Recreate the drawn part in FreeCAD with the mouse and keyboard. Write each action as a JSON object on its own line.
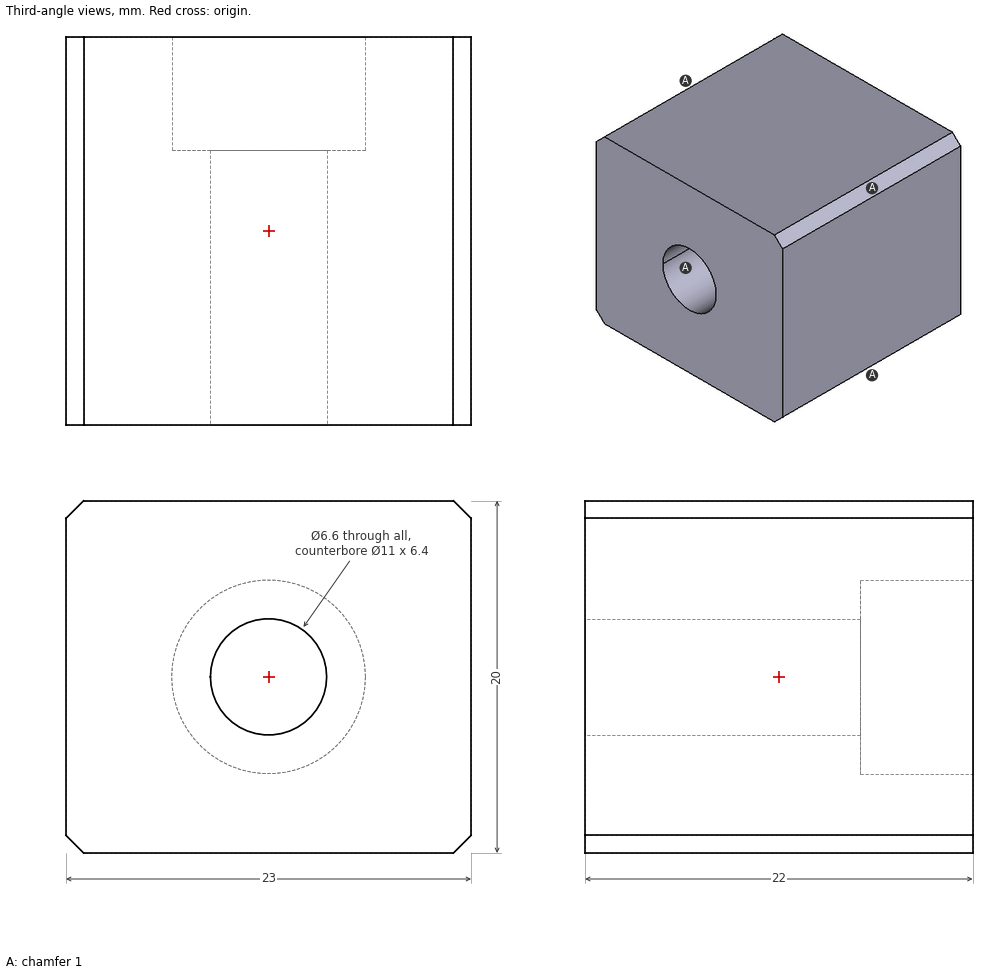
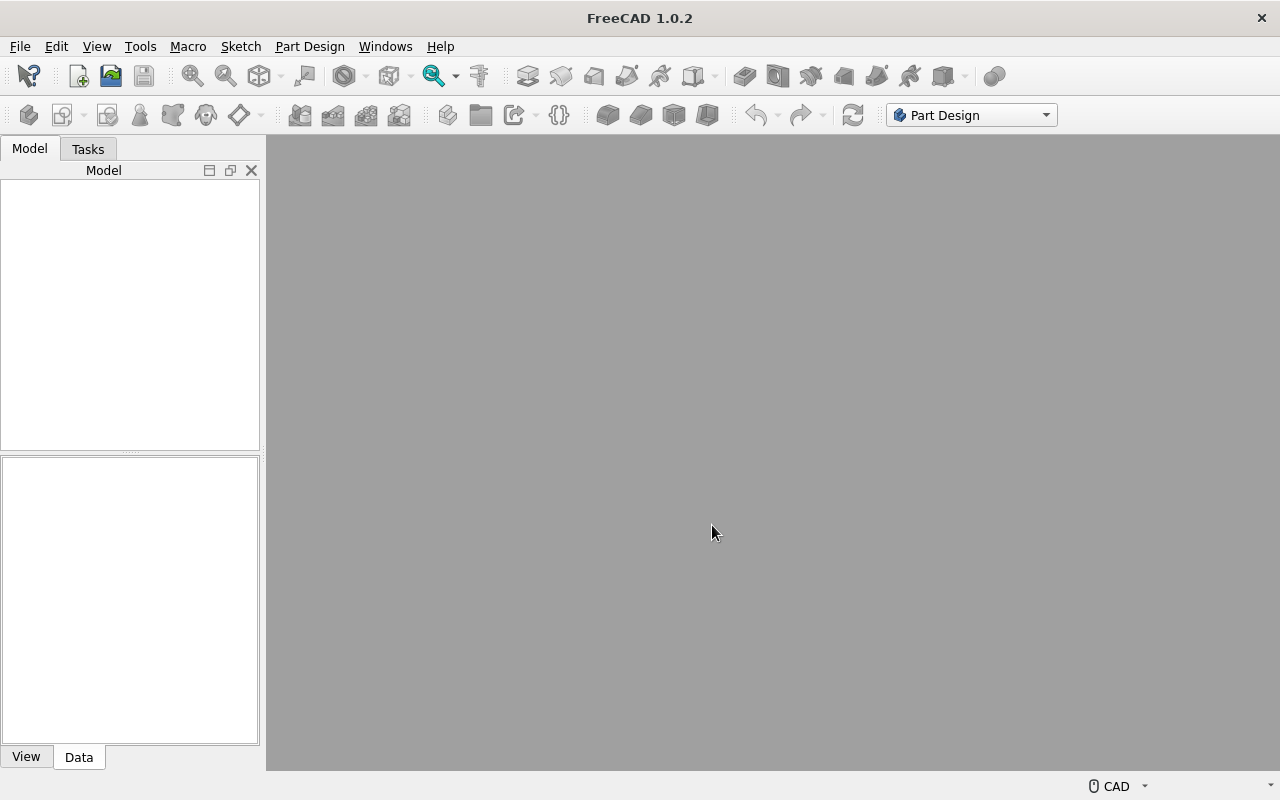
{"action": "left_click", "coordinate": [78, 76]}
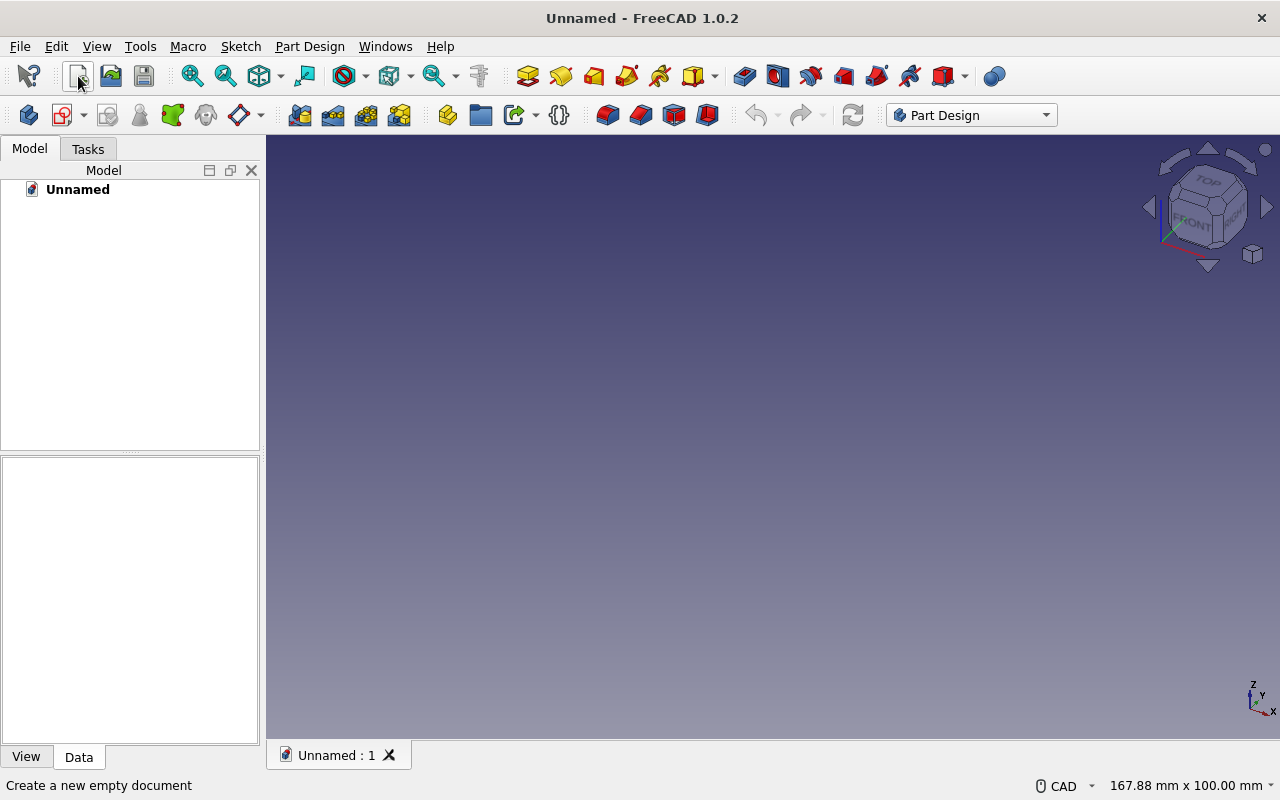
{"action": "left_click", "coordinate": [62, 116]}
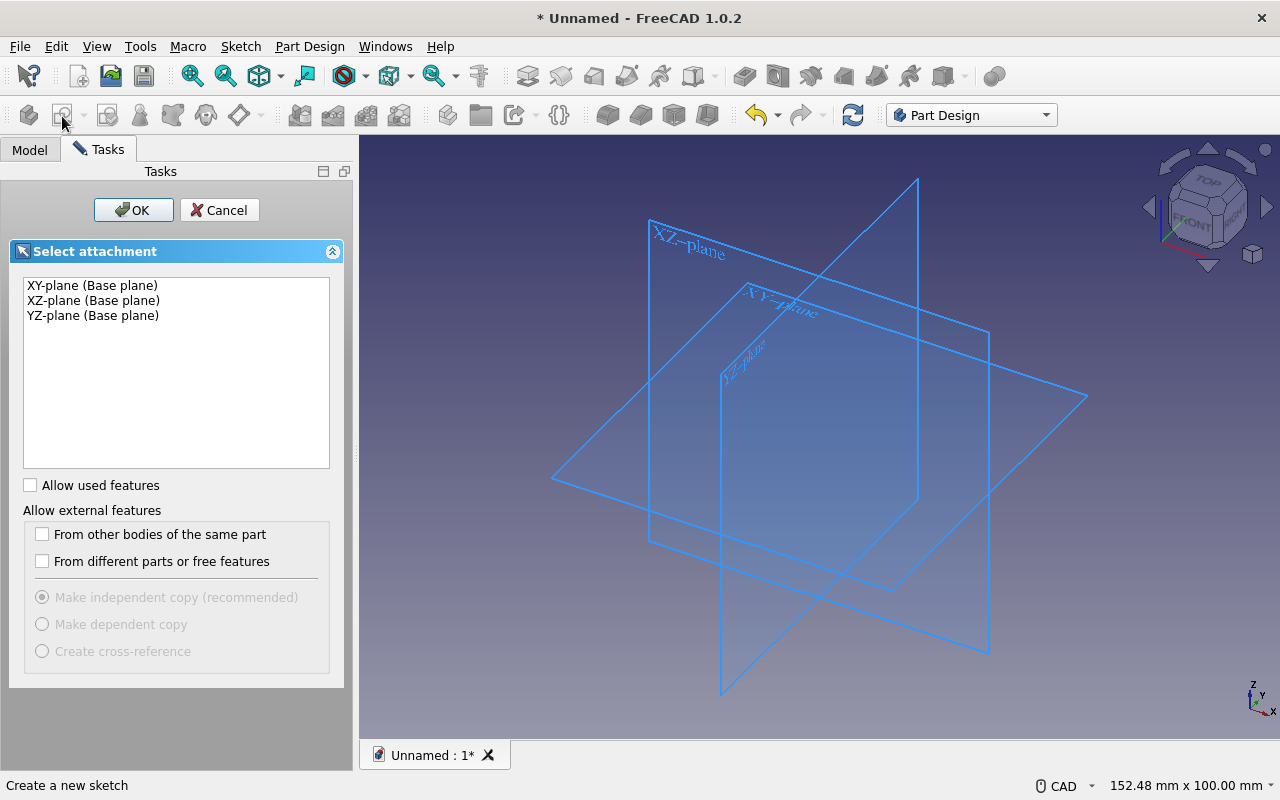
{"action": "left_click", "coordinate": [84, 300]}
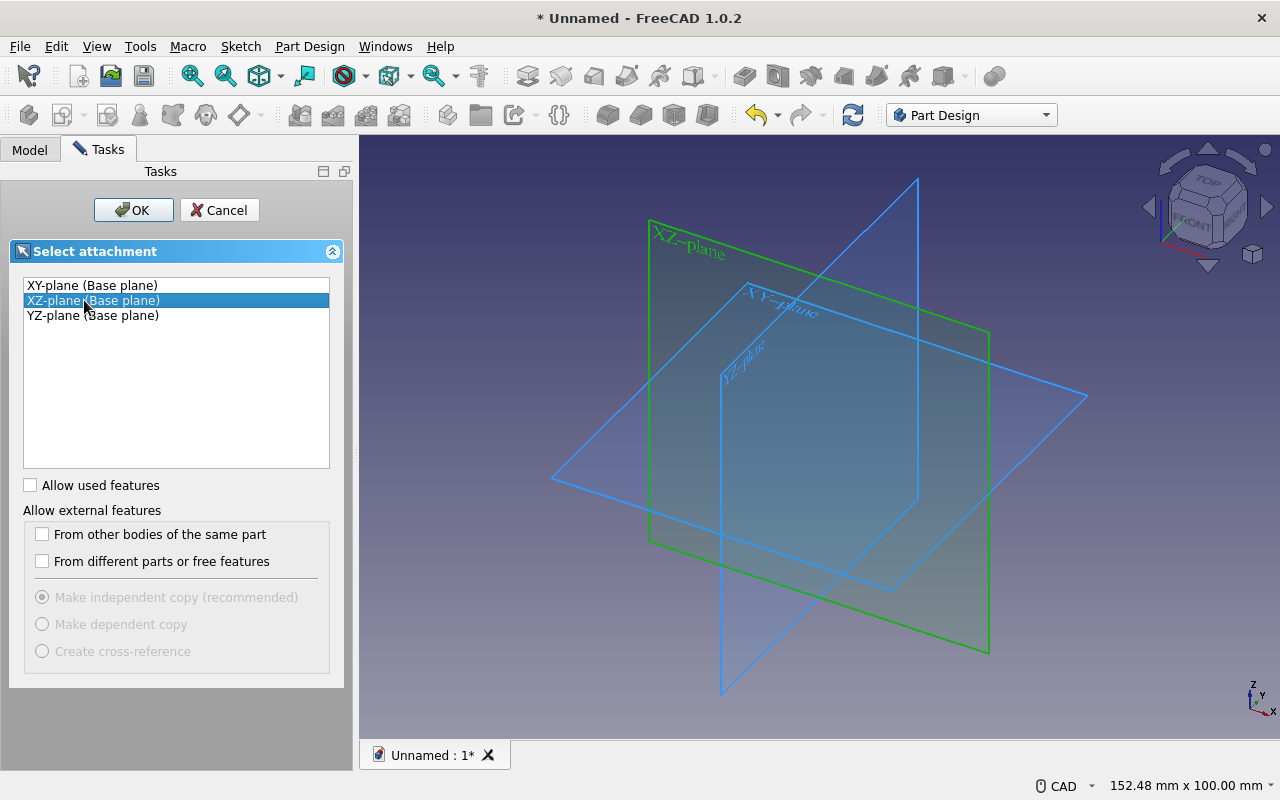
{"action": "left_click", "coordinate": [134, 210]}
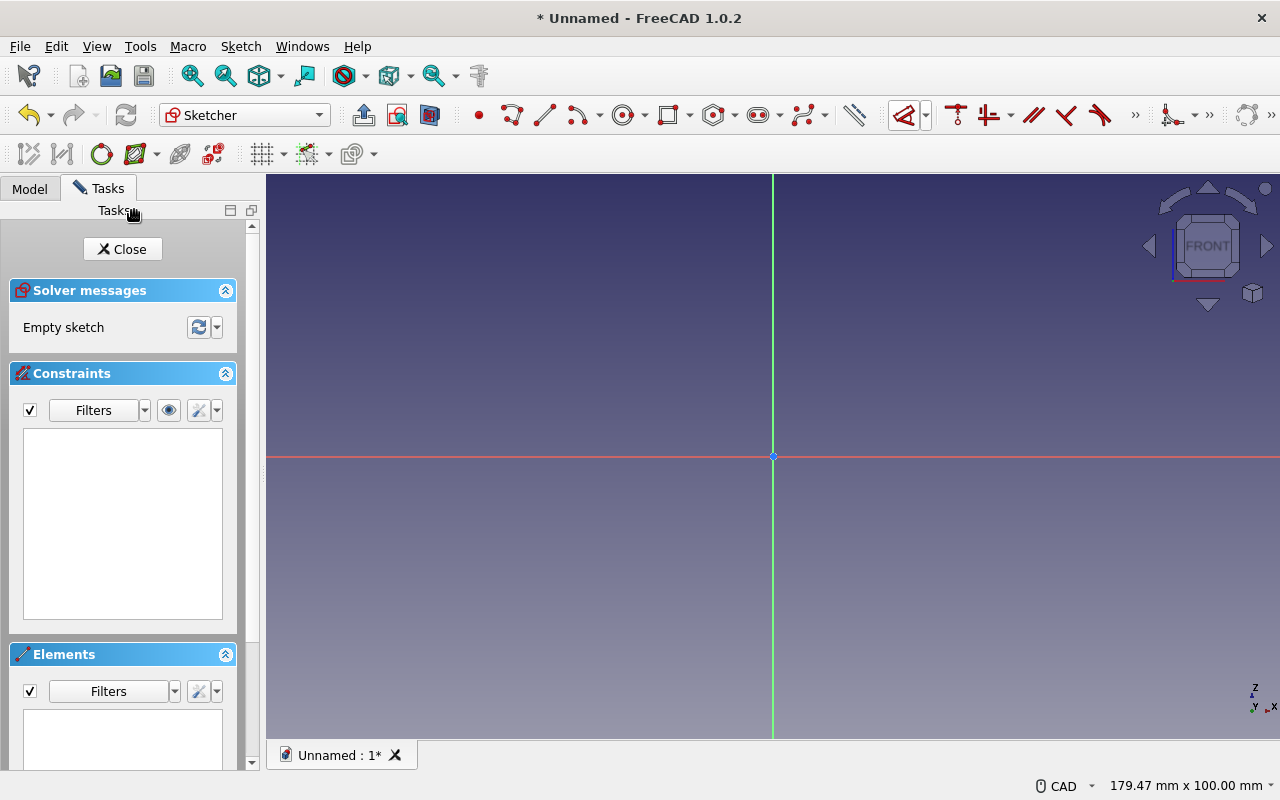
{"action": "scroll", "coordinate": [803, 456], "scroll_direction": "up", "scroll_amount": 6}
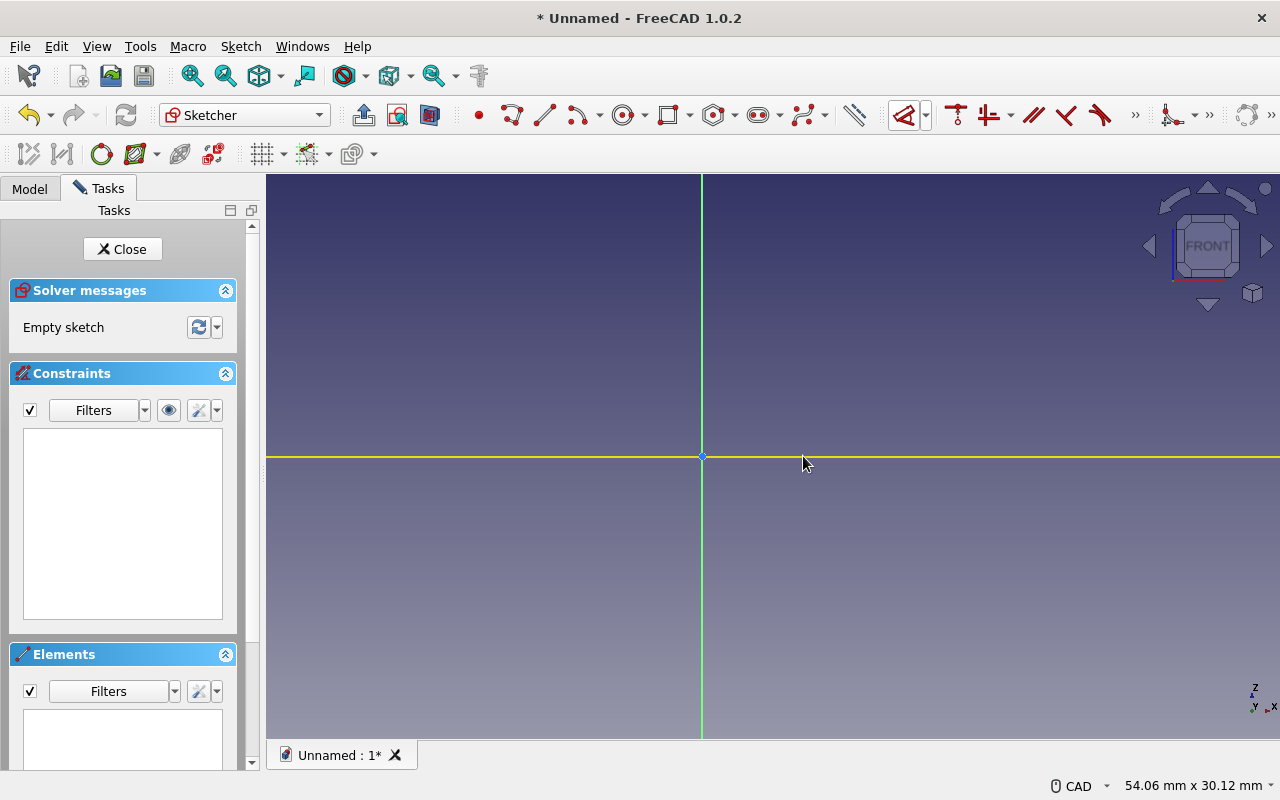
{"action": "key", "text": "g v"}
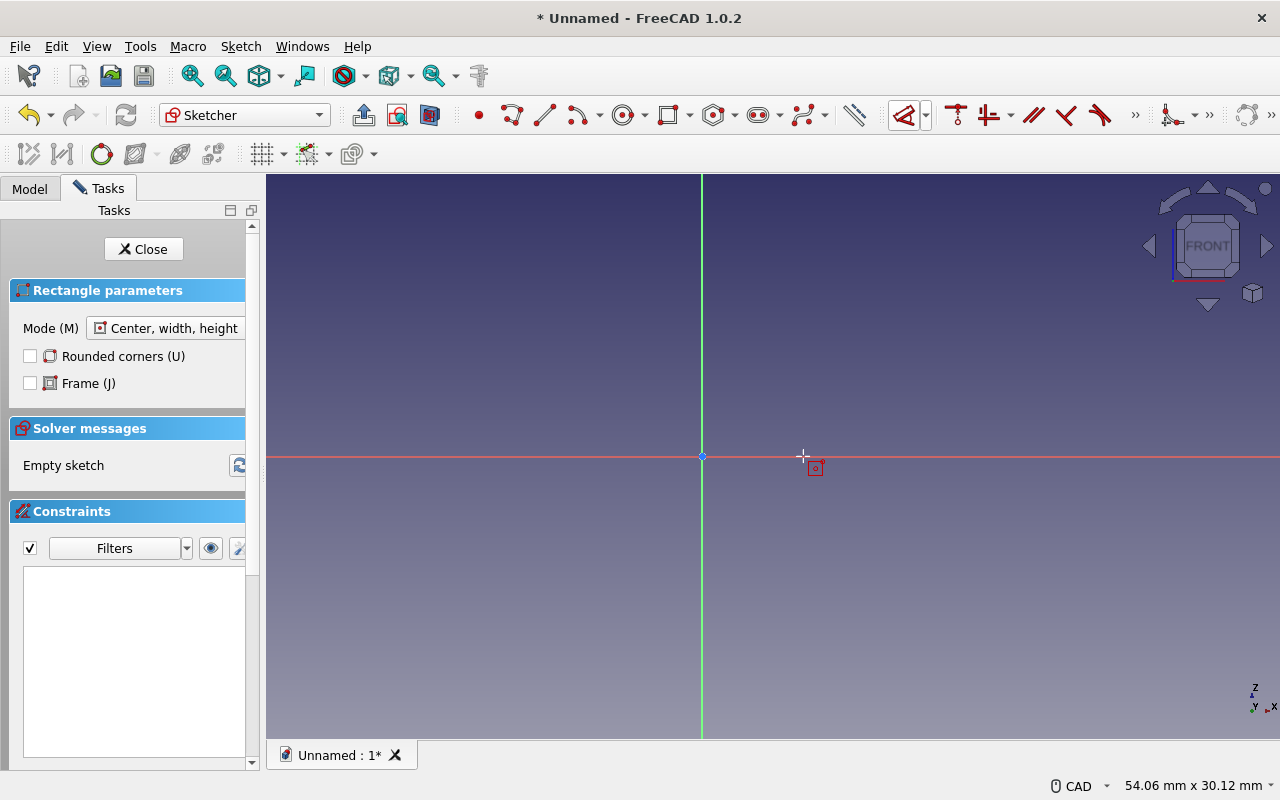
{"action": "left_click", "coordinate": [702, 456]}
{"action": "left_click", "coordinate": [918, 269]}
{"action": "key", "text": "Escape"}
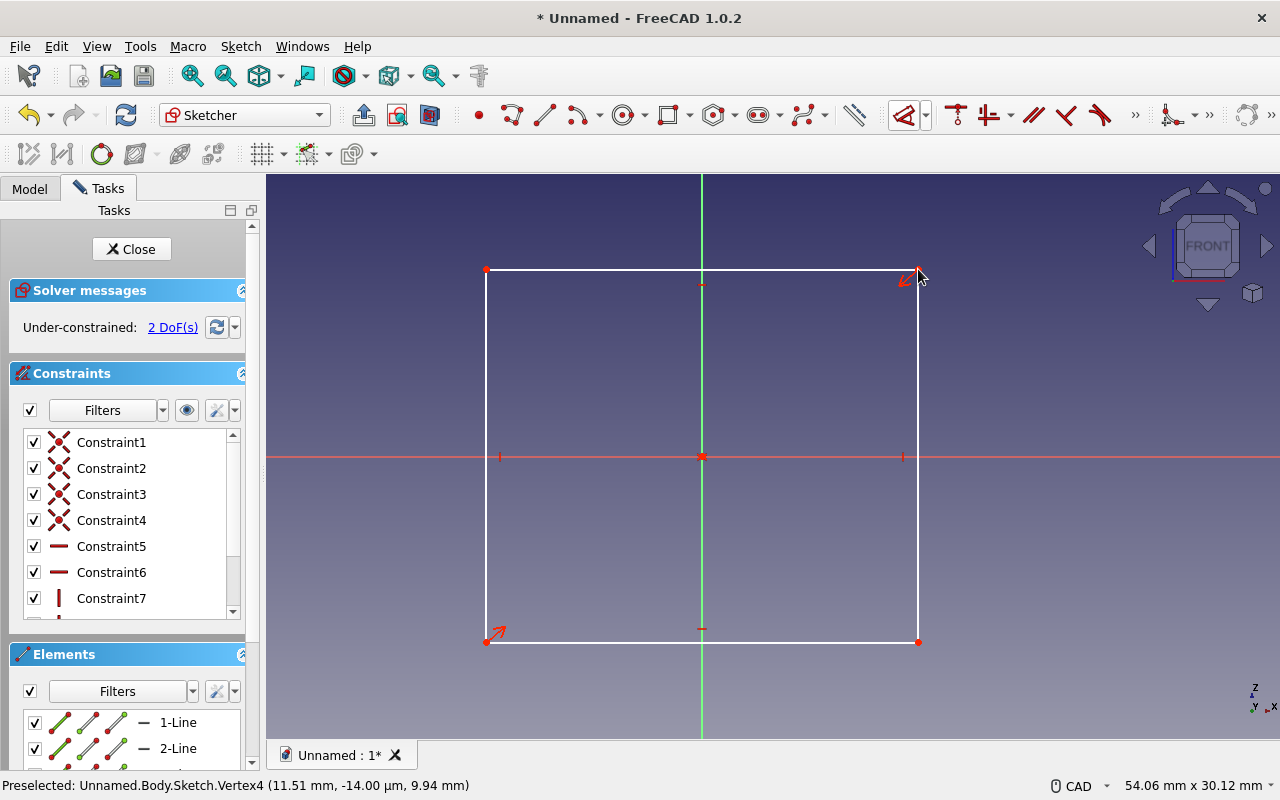
{"action": "key", "text": "d"}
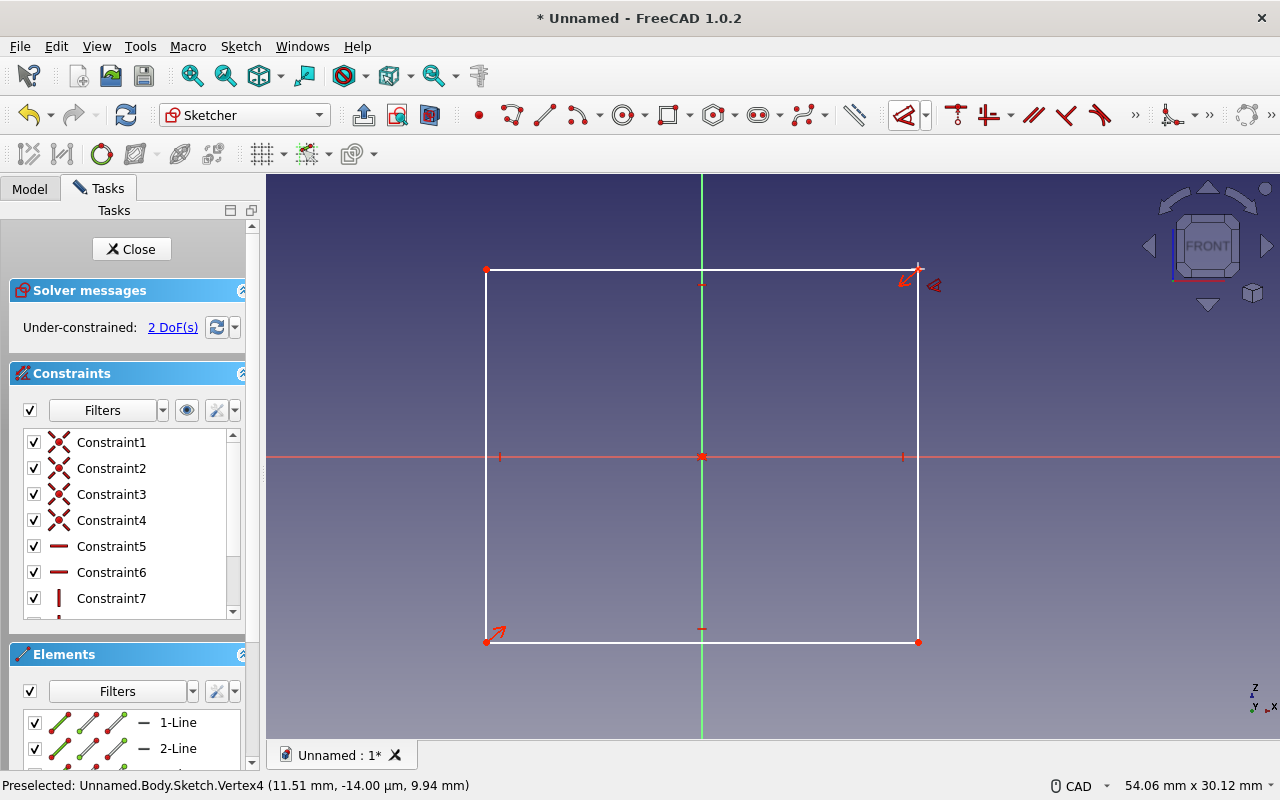
{"action": "left_click", "coordinate": [616, 643]}
{"action": "left_click", "coordinate": [603, 677]}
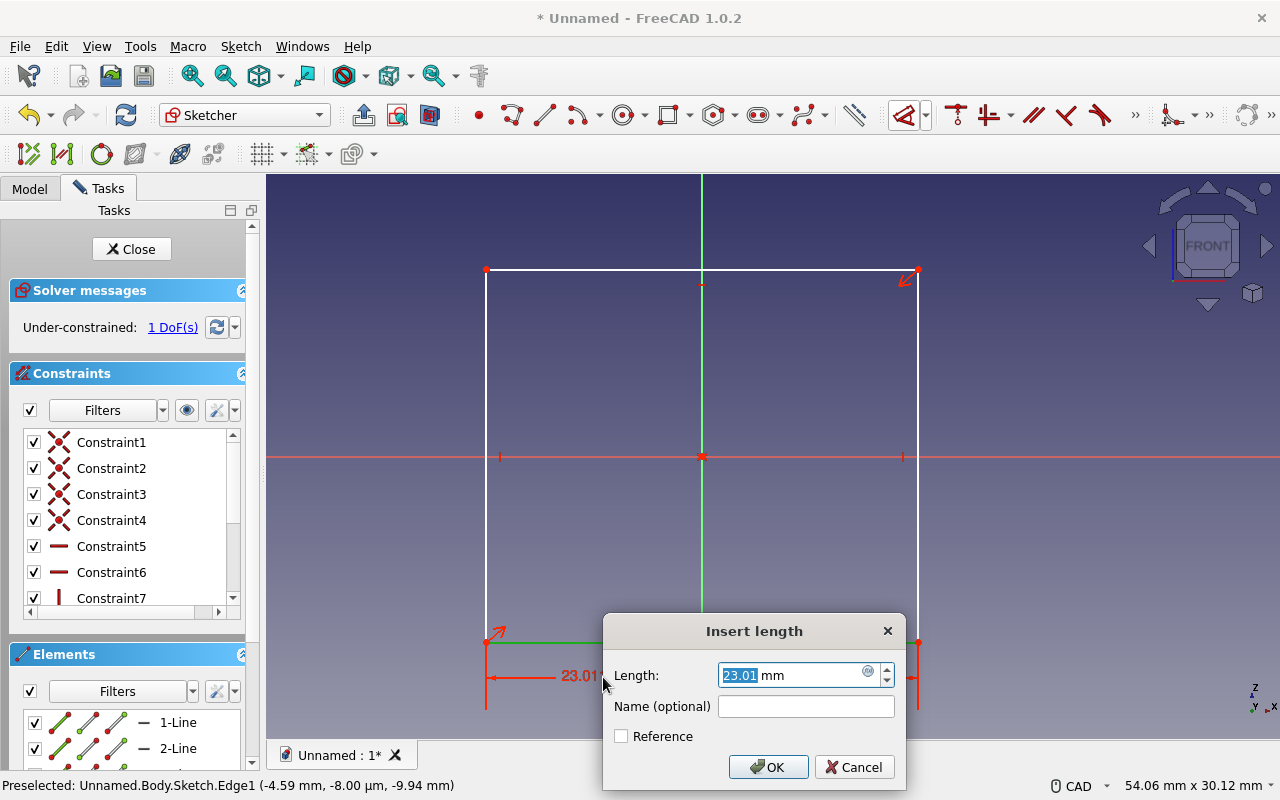
{"action": "type", "text": "23"}
{"action": "key", "text": "Return"}